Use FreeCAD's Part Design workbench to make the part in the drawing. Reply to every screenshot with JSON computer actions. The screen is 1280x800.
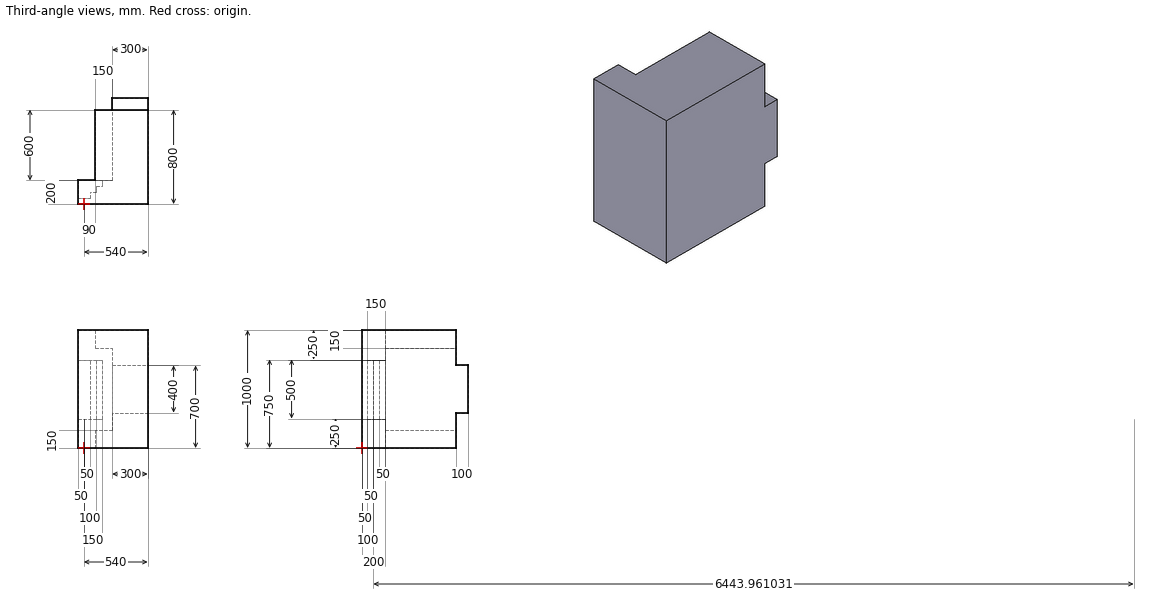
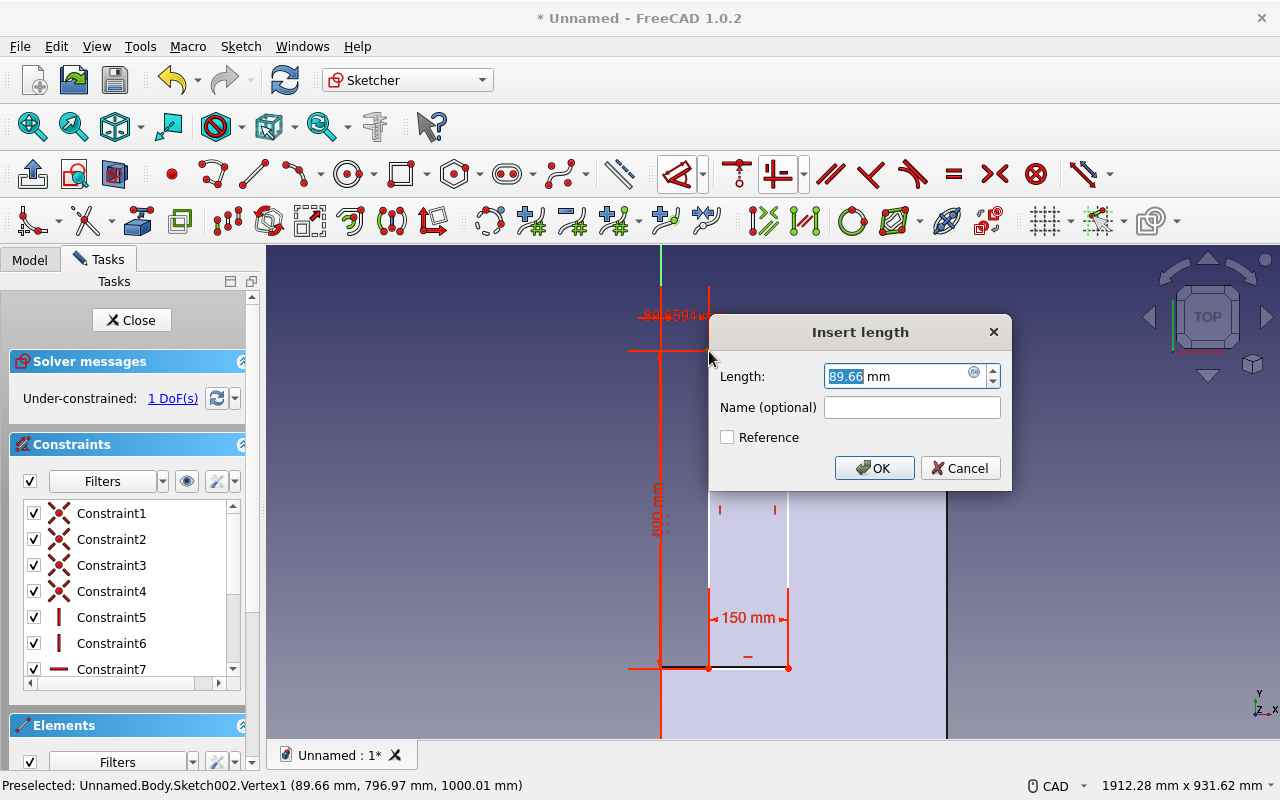
{"action": "type", "text": "90"}
{"action": "key", "text": "Return"}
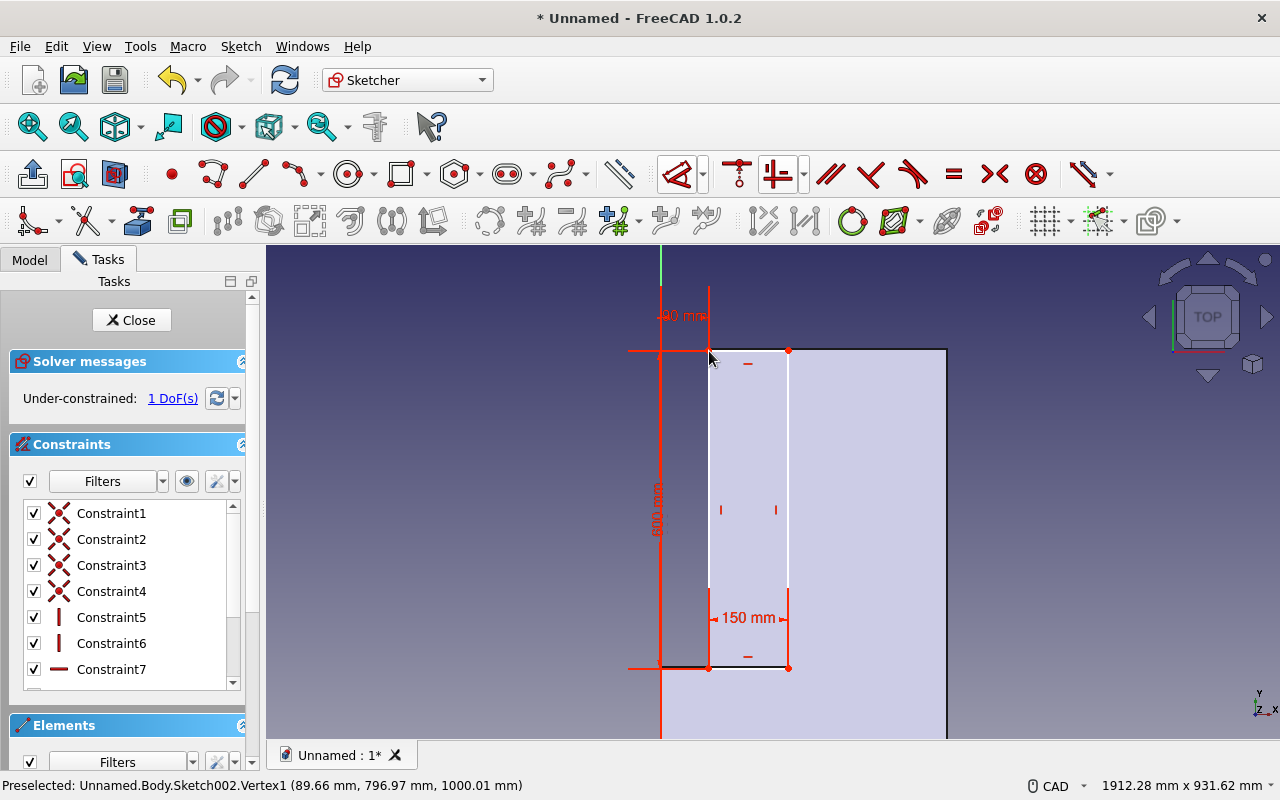
{"action": "left_click", "coordinate": [709, 351]}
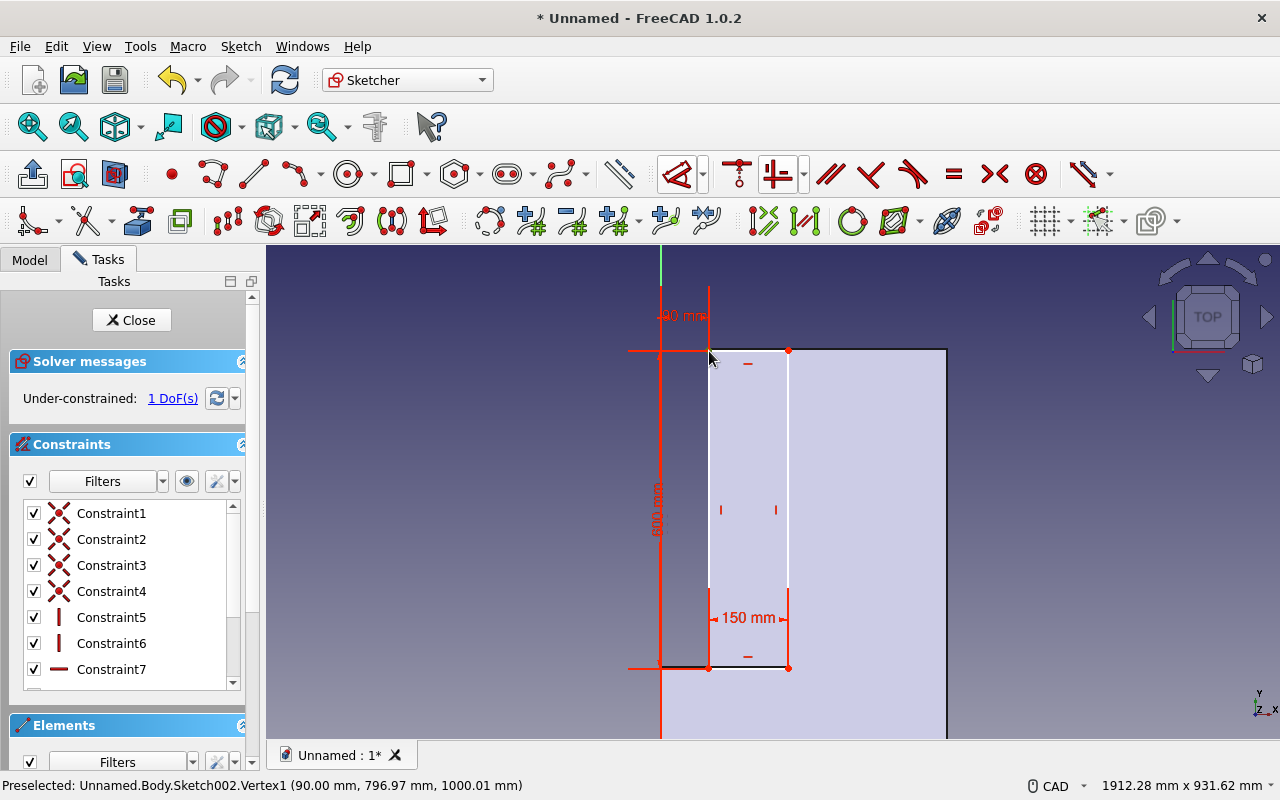
{"action": "left_click", "coordinate": [702, 174]}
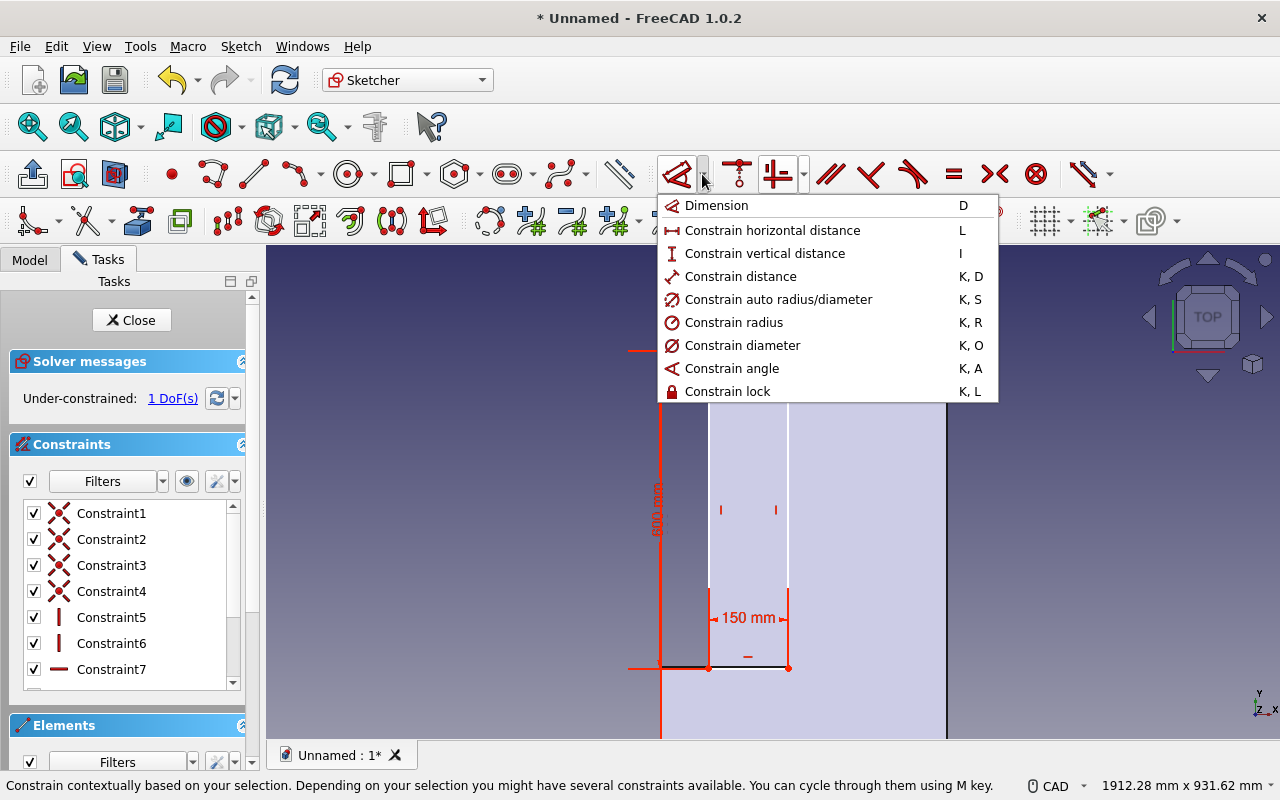
{"action": "left_click", "coordinate": [828, 254]}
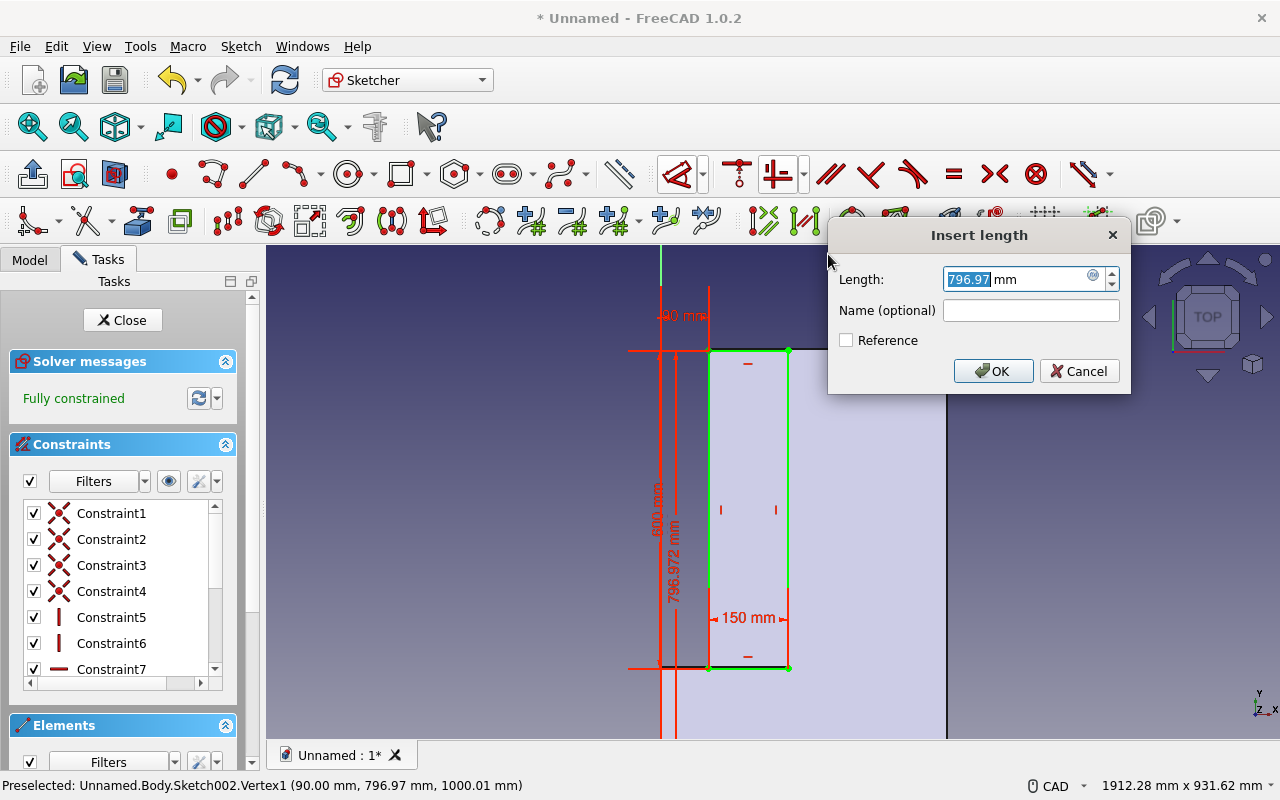
{"action": "type", "text": "800"}
{"action": "key", "text": "Return"}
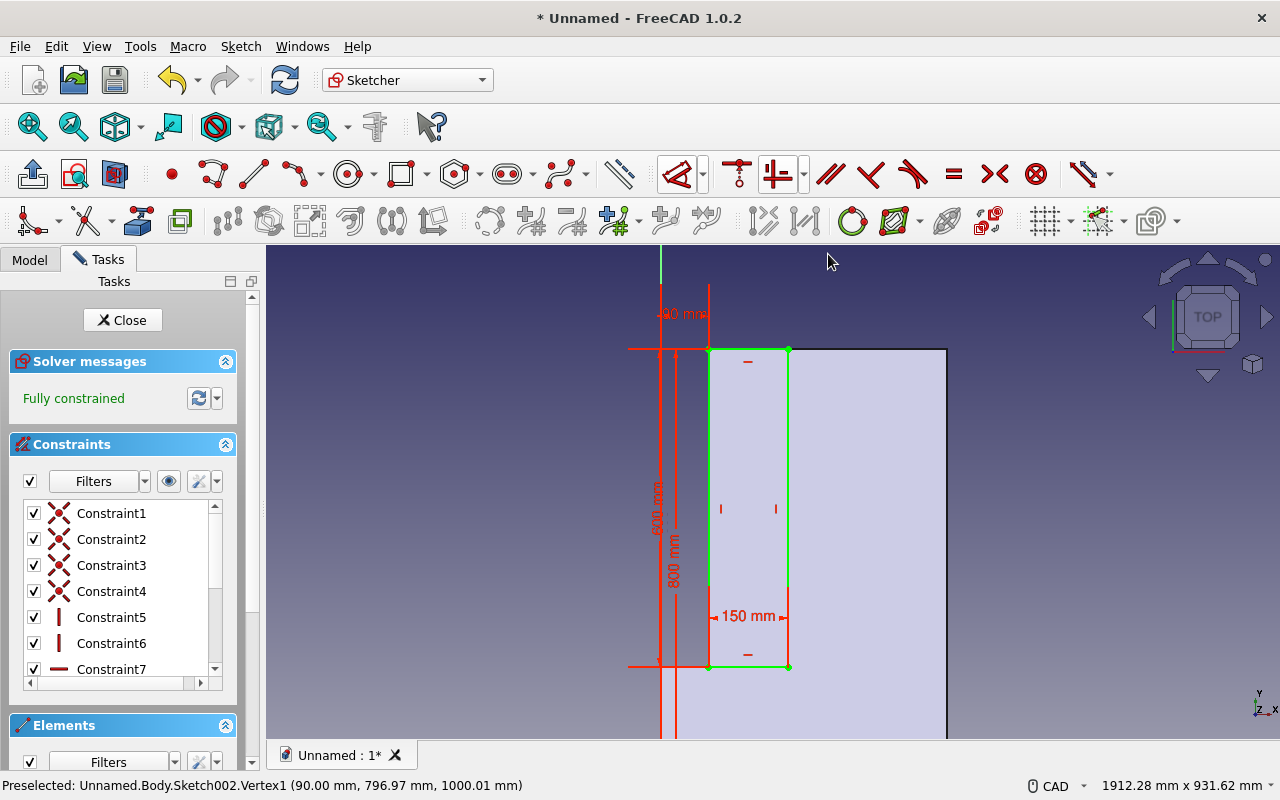
{"action": "left_click", "coordinate": [123, 320]}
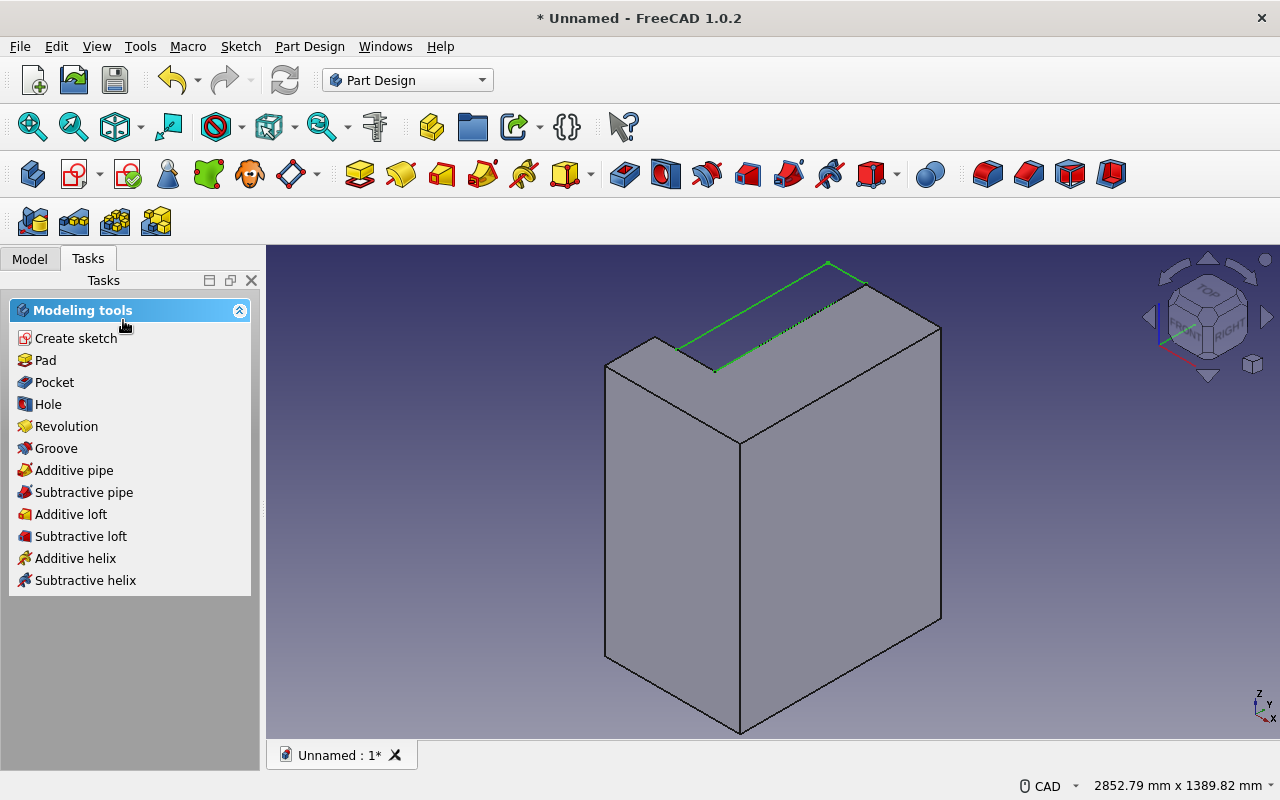
{"action": "left_click", "coordinate": [360, 174]}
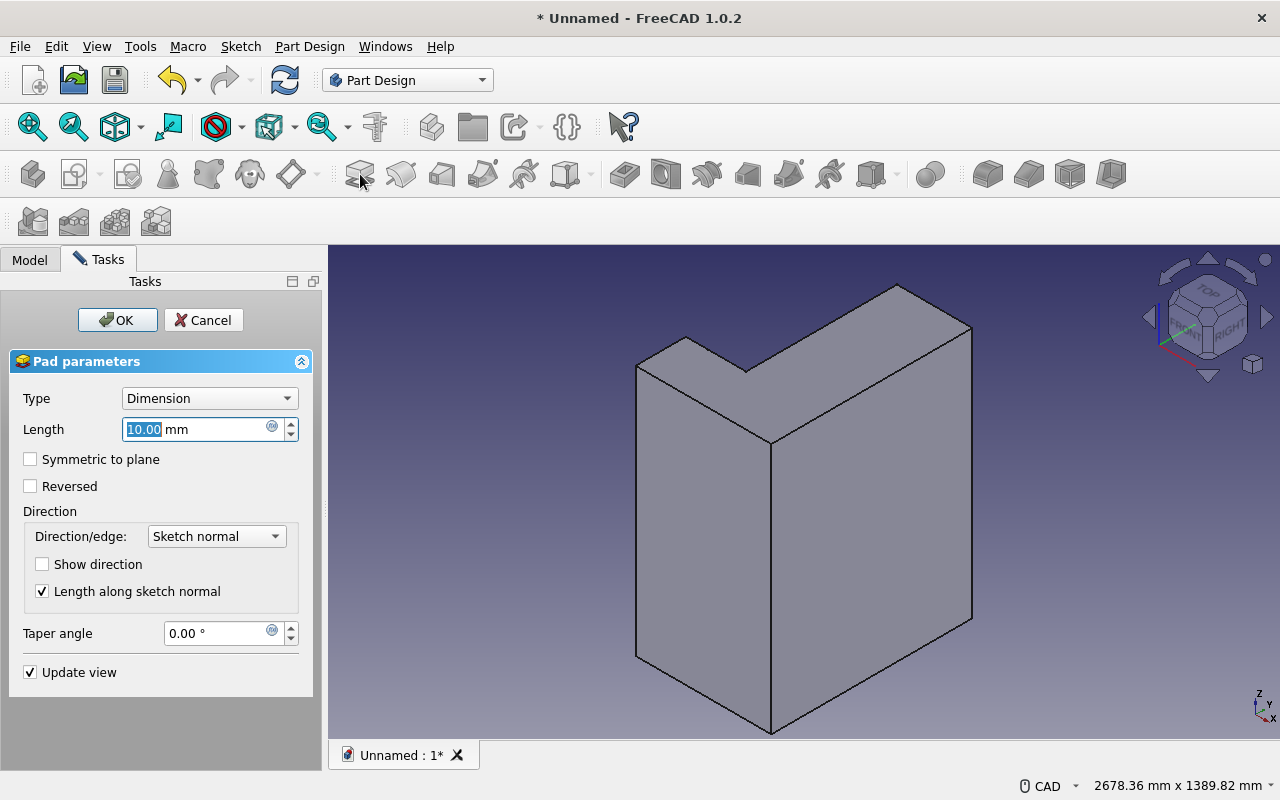
{"action": "type", "text": "150"}
{"action": "key", "text": "Tab"}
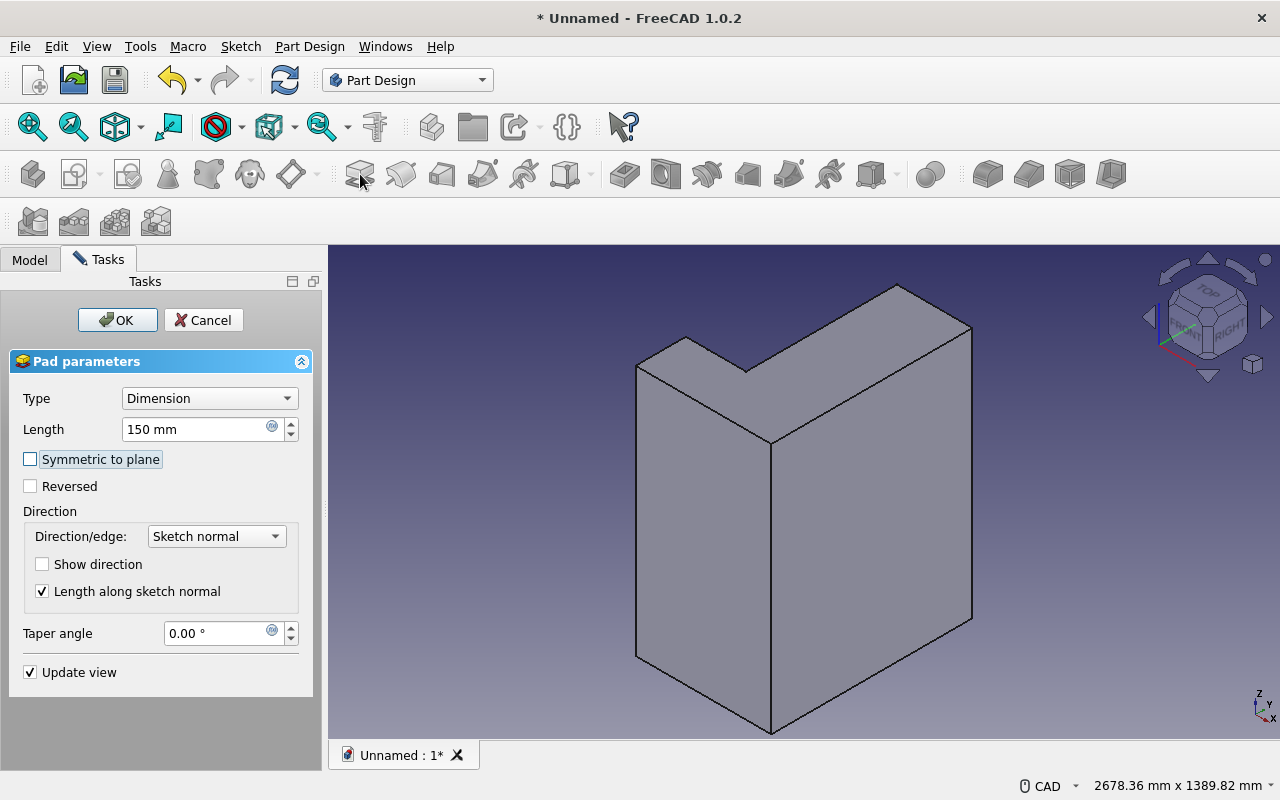
{"action": "left_click", "coordinate": [31, 486]}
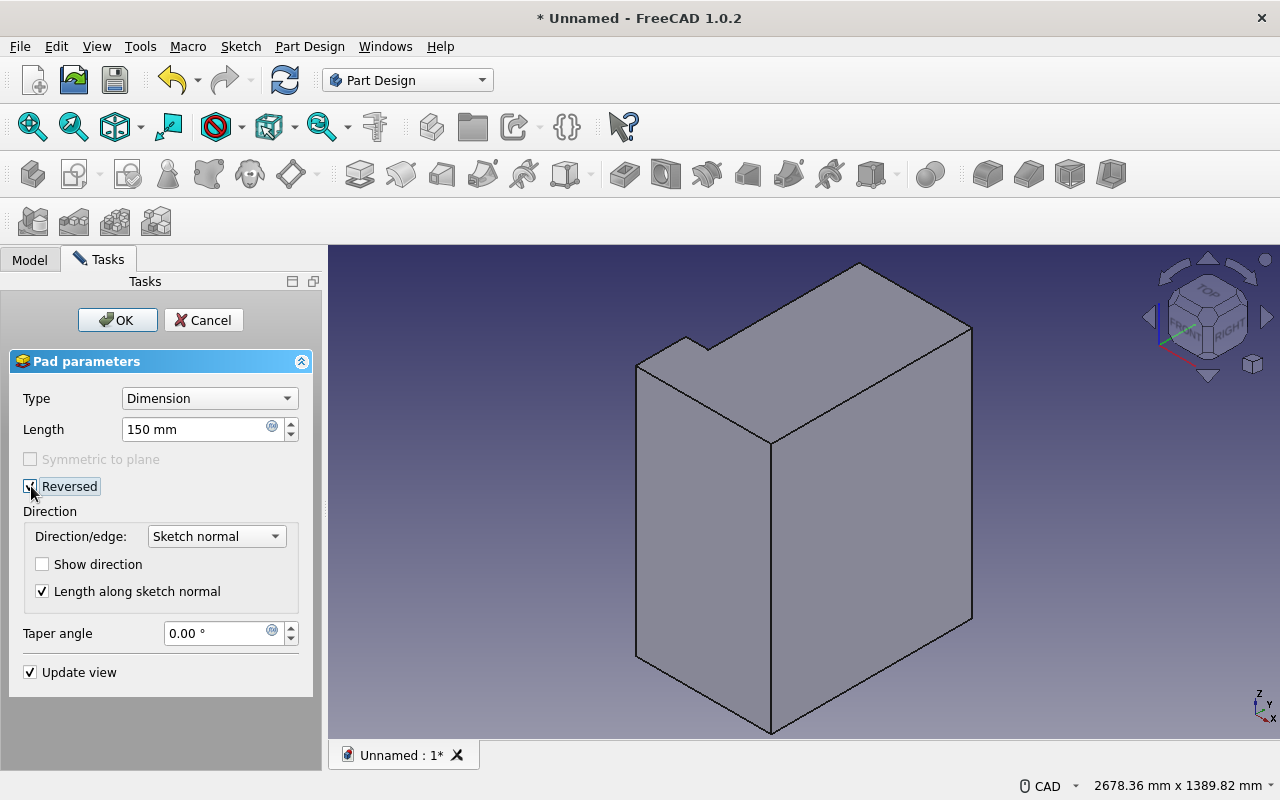
{"action": "left_click", "coordinate": [118, 320]}